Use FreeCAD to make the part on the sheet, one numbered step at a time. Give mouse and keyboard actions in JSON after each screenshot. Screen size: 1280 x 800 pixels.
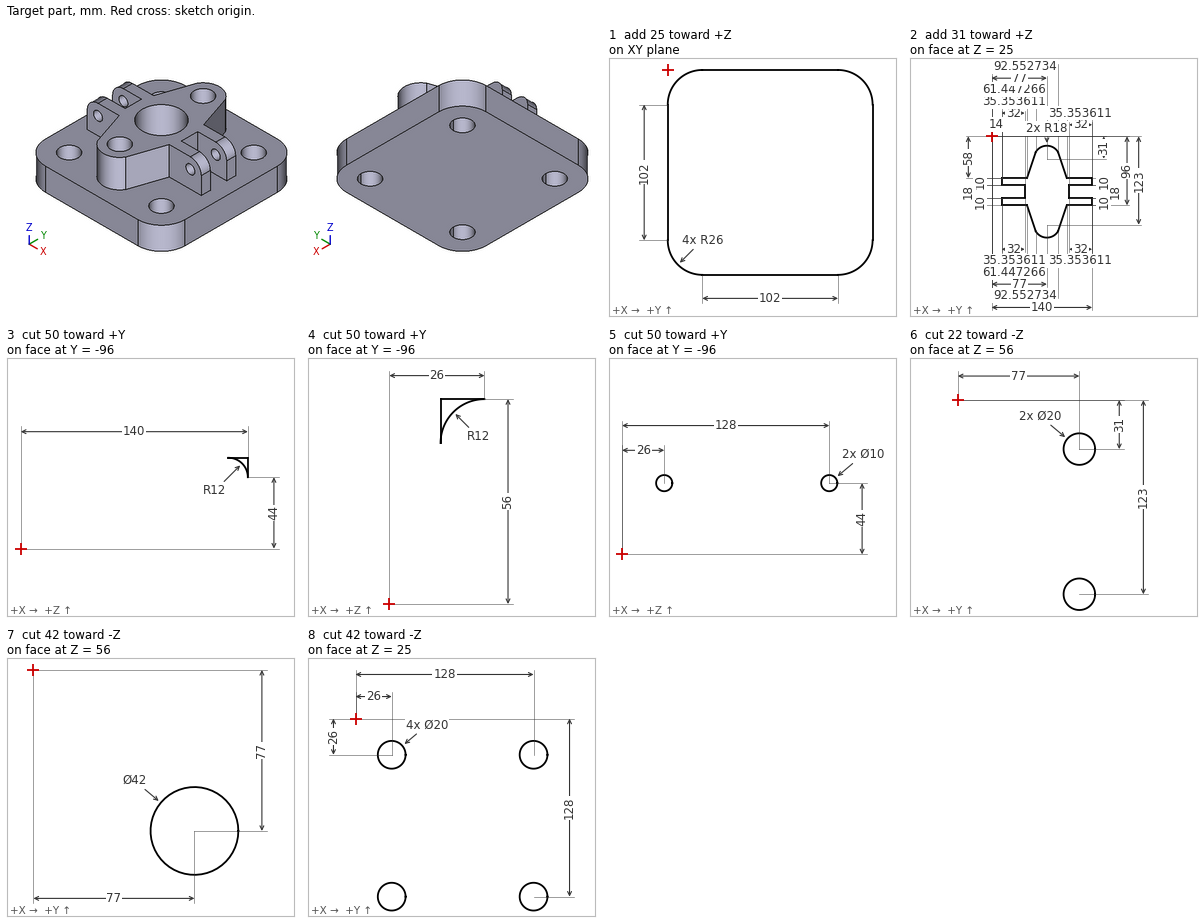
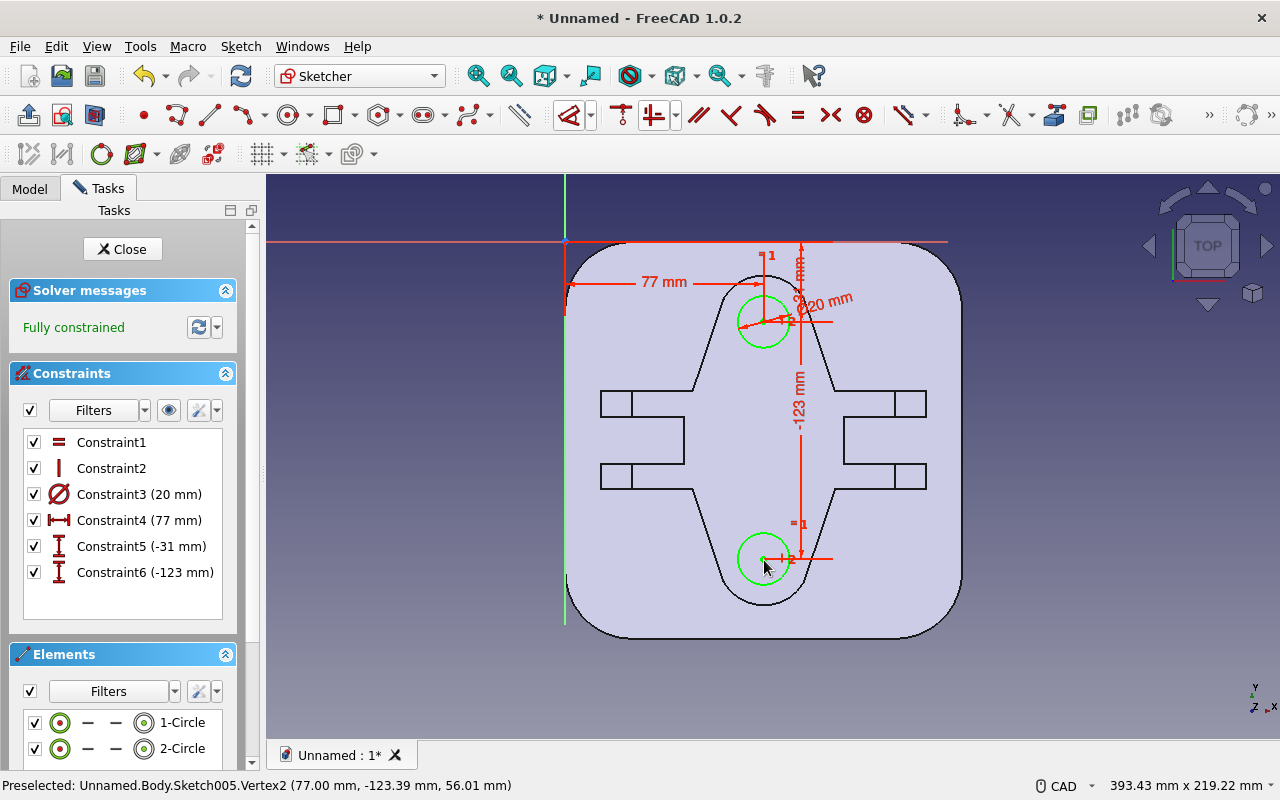
{"action": "left_click", "coordinate": [123, 249]}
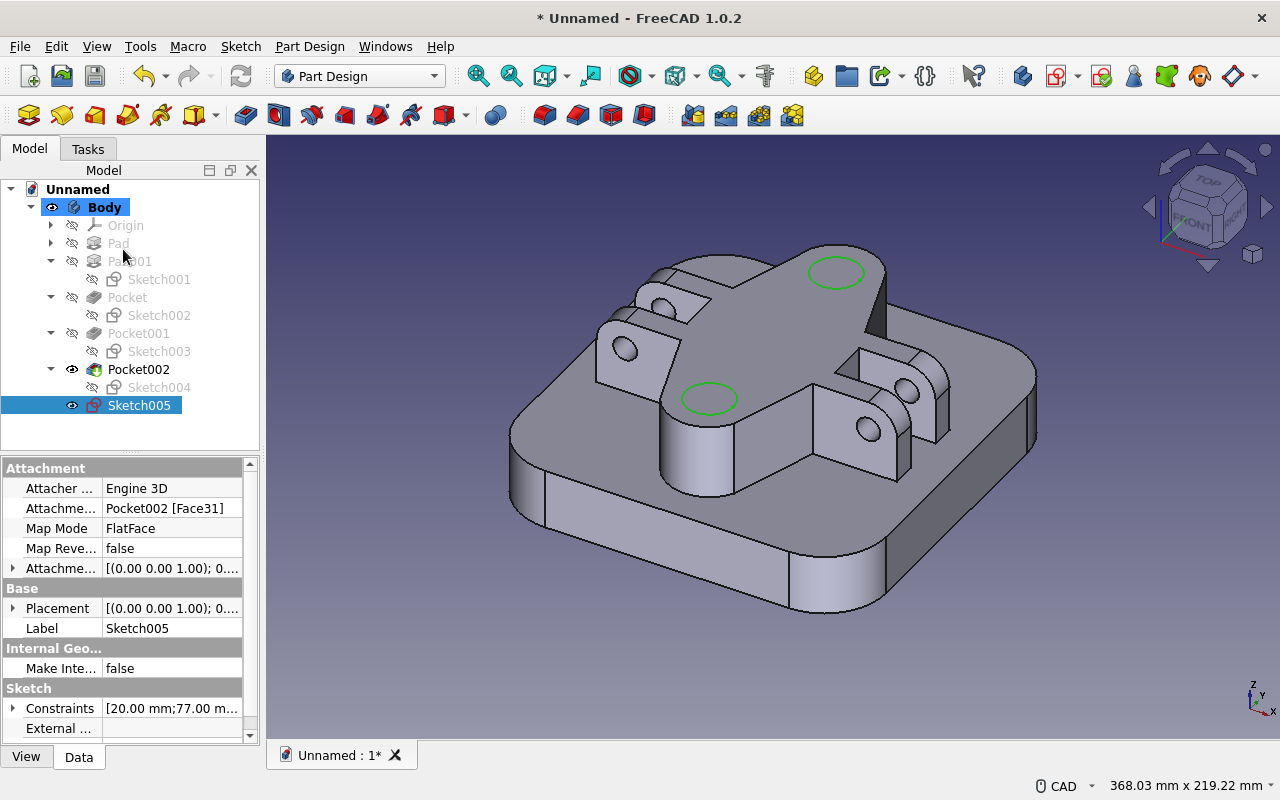
{"action": "left_click", "coordinate": [246, 116]}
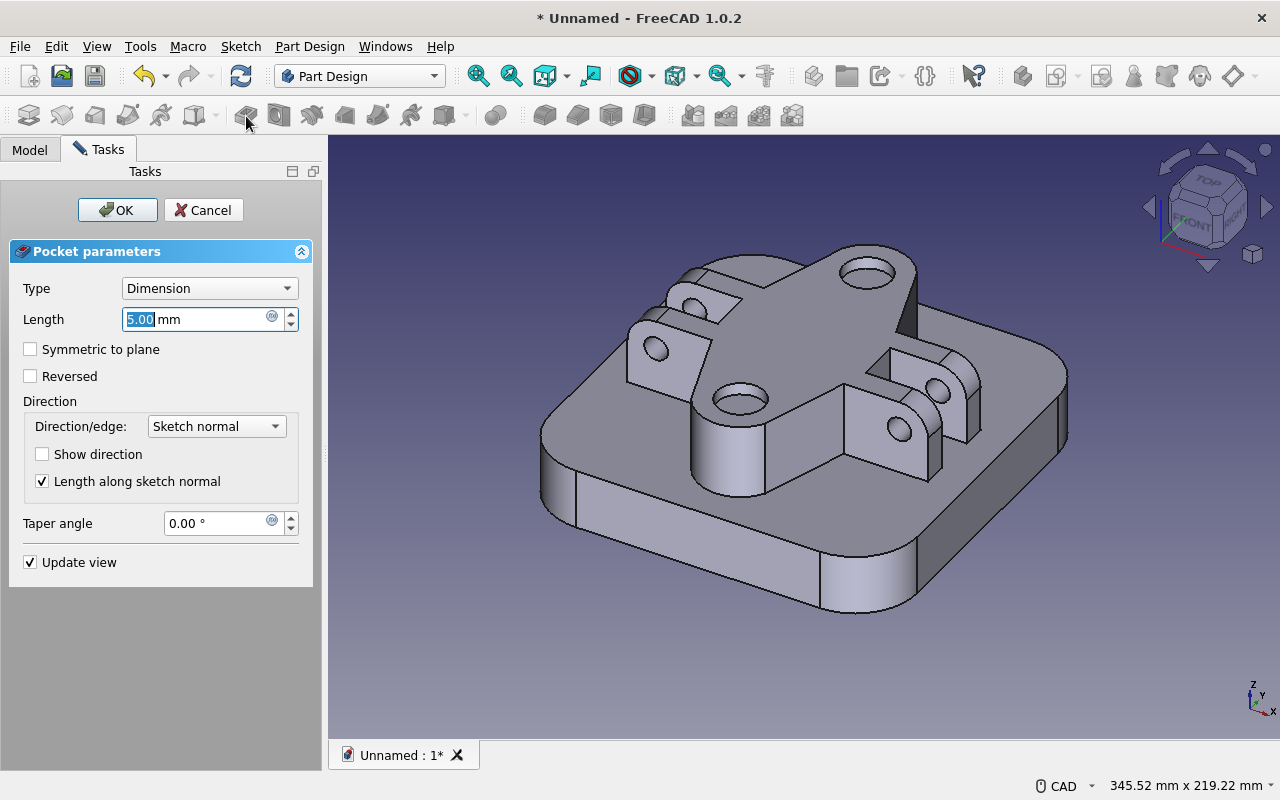
{"action": "type", "text": "22"}
{"action": "key", "text": "Tab"}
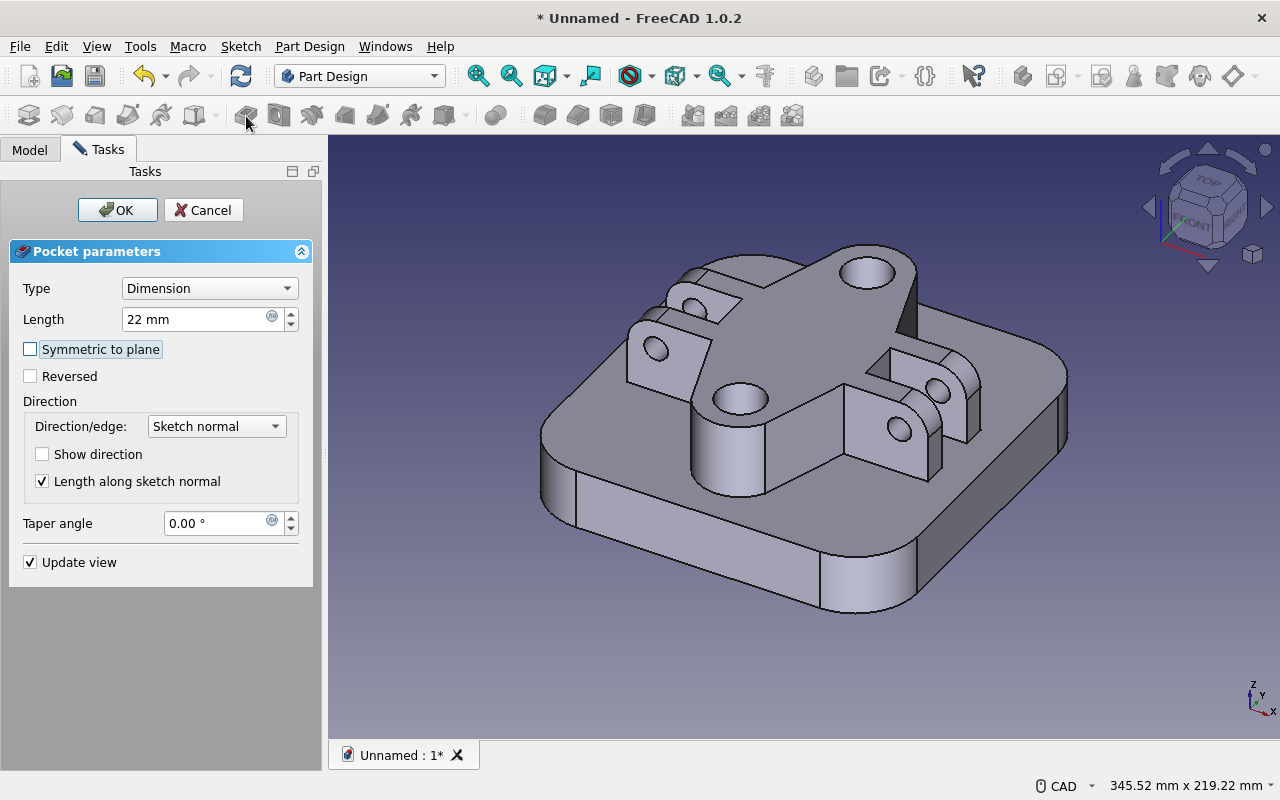
{"action": "left_click", "coordinate": [118, 210]}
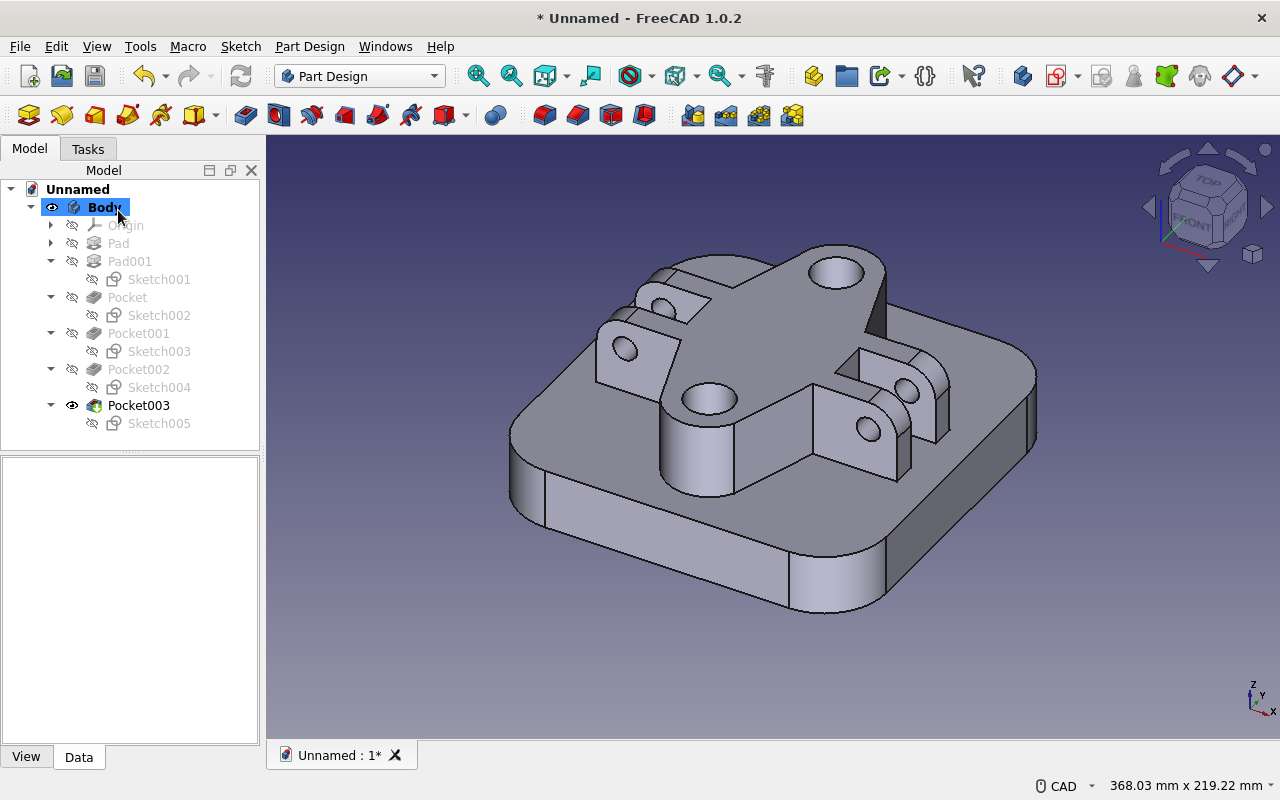
{"action": "left_click", "coordinate": [773, 335]}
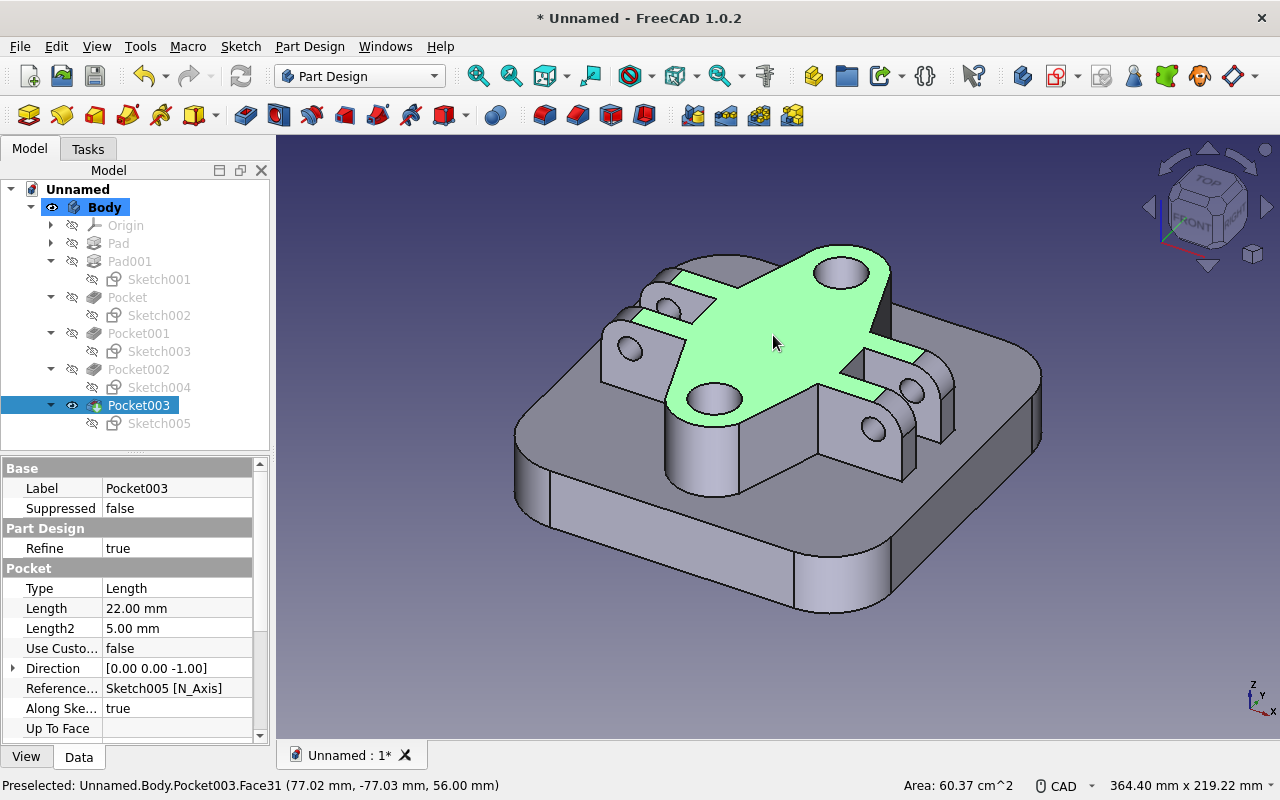
{"action": "left_click", "coordinate": [1056, 76]}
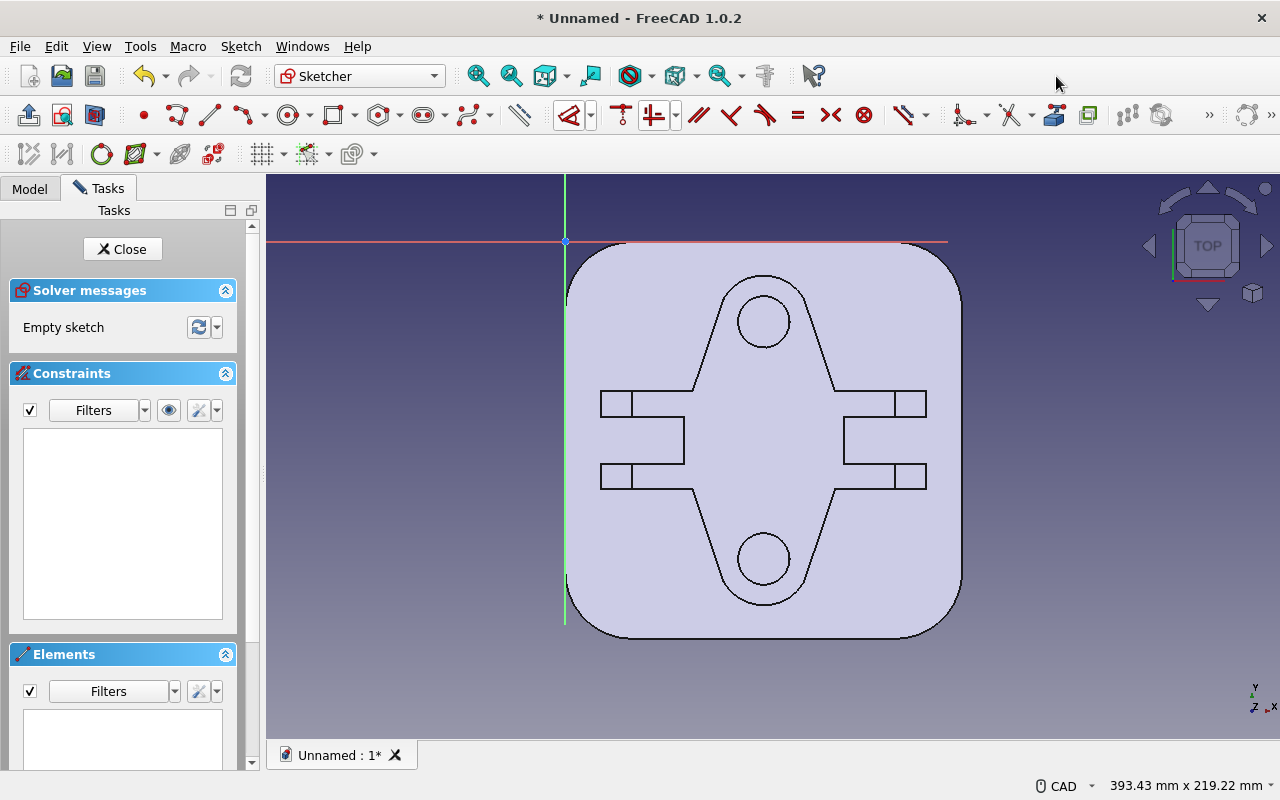
{"action": "scroll", "coordinate": [665, 202], "scroll_direction": "up", "scroll_amount": 2}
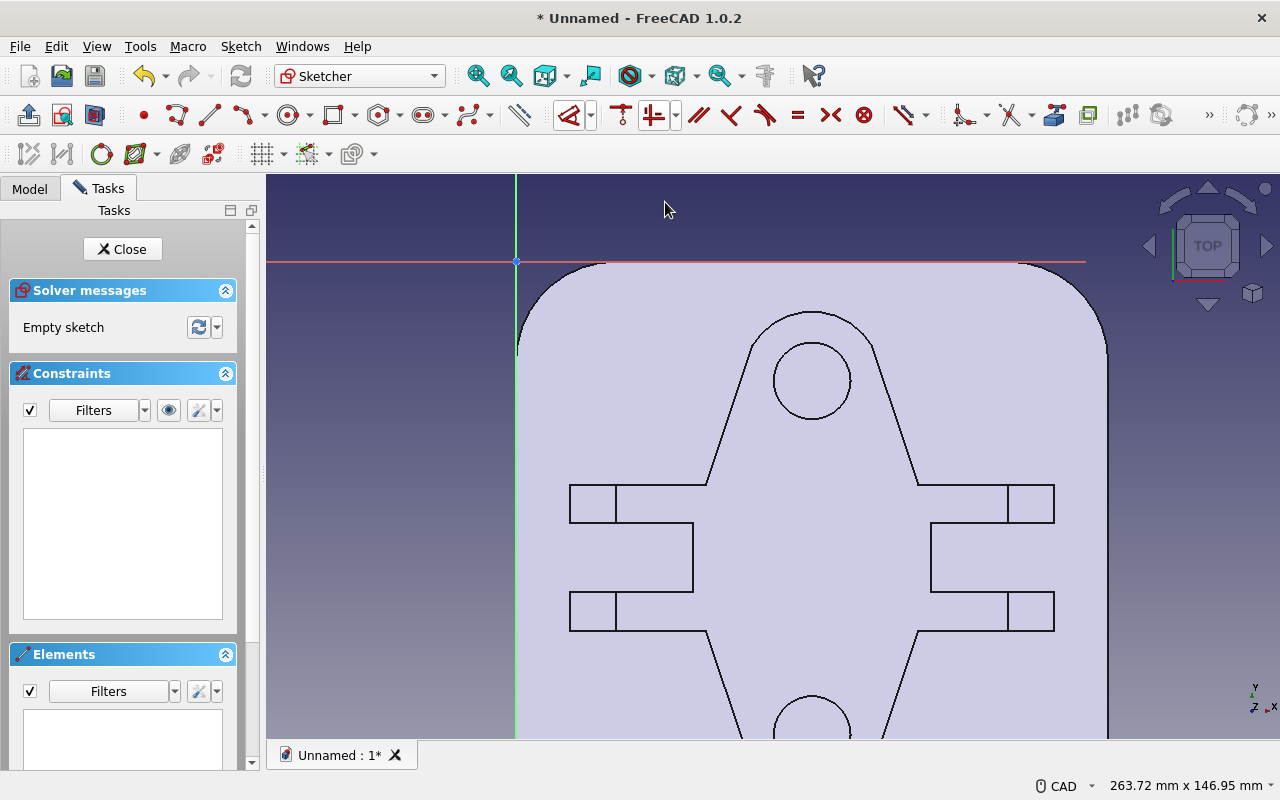
{"action": "left_click", "coordinate": [288, 116]}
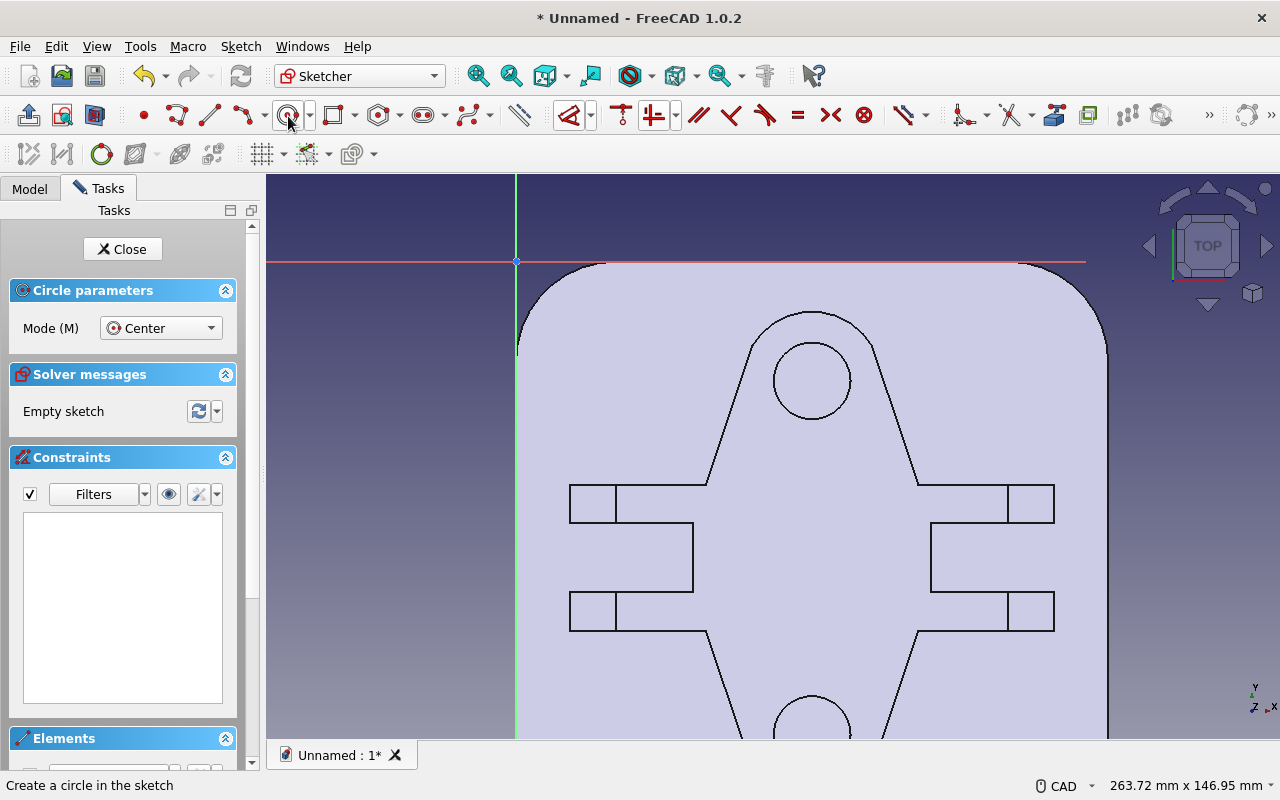
{"action": "left_click", "coordinate": [812, 558]}
{"action": "left_click", "coordinate": [869, 501]}
{"action": "key", "text": "Escape"}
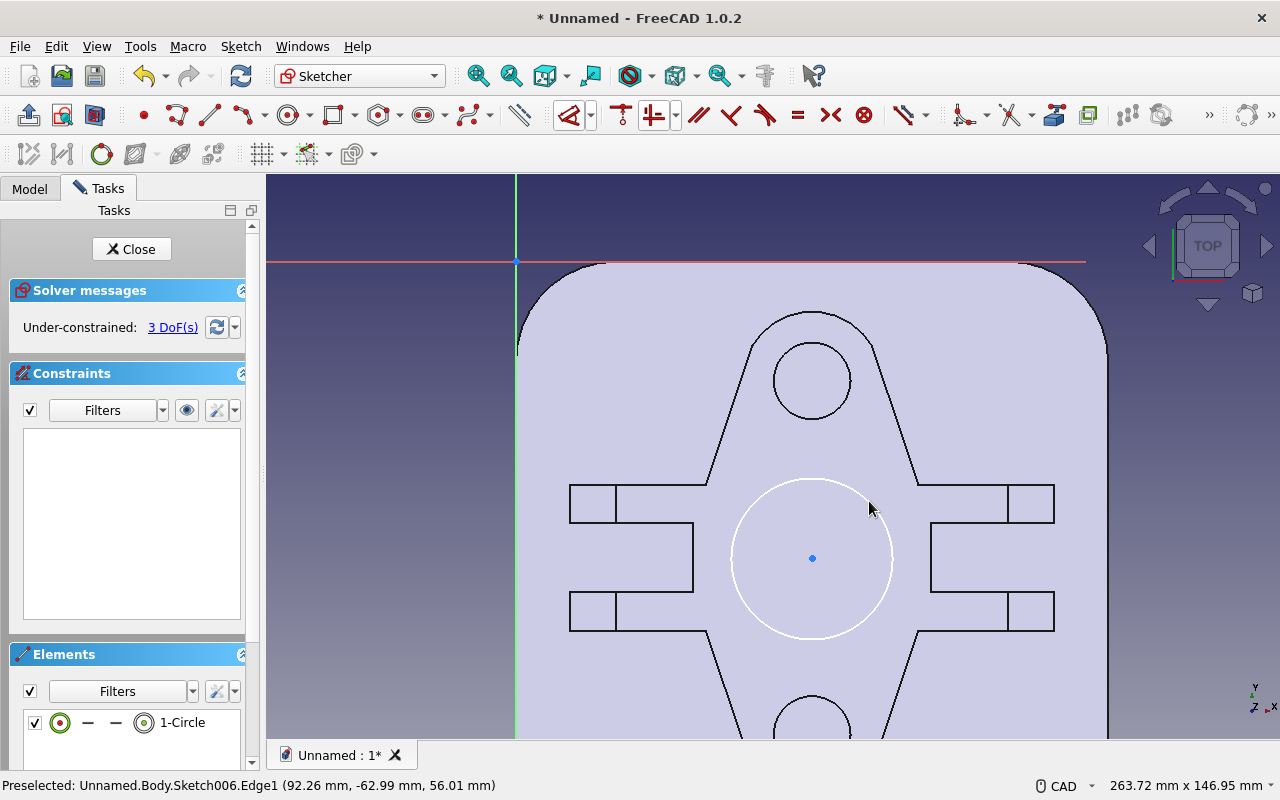
{"action": "left_click", "coordinate": [869, 502]}